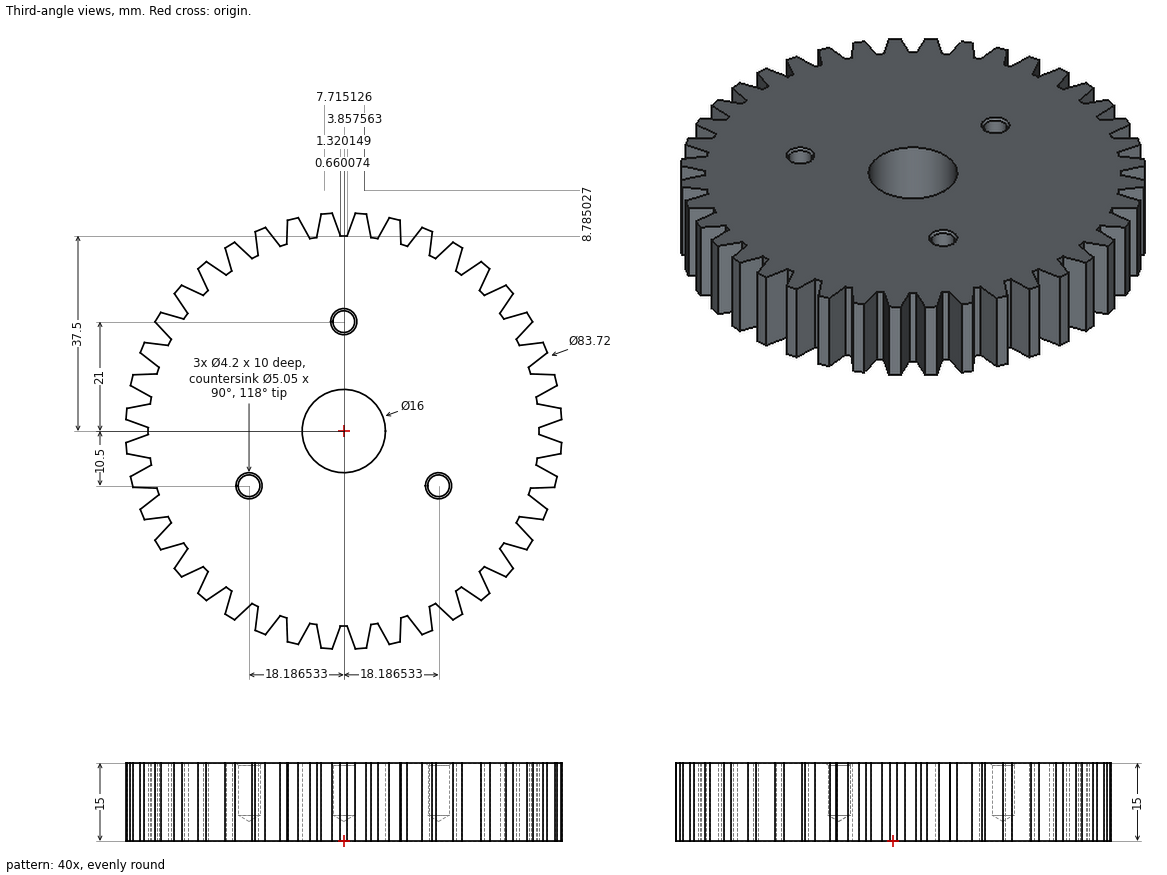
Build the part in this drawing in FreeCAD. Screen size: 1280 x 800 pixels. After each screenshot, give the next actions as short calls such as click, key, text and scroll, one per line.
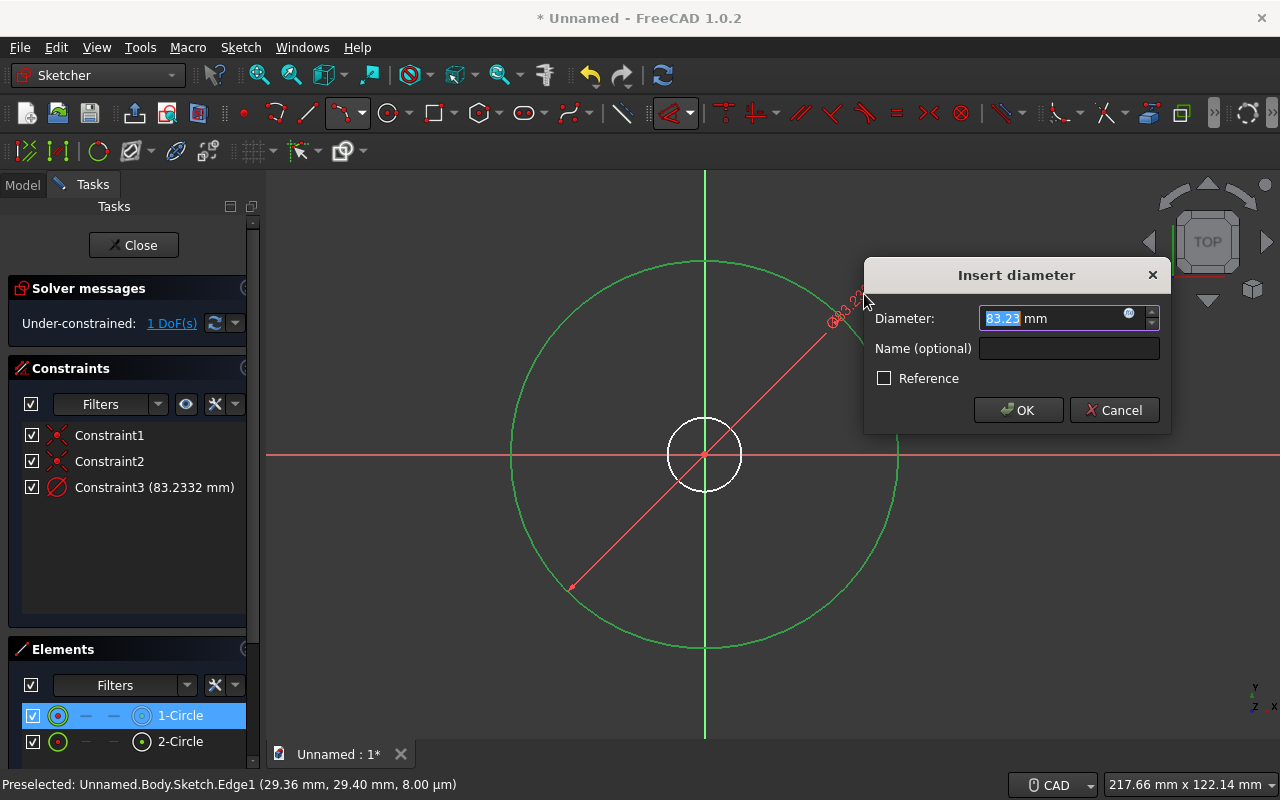
text(83.72)
key(Return)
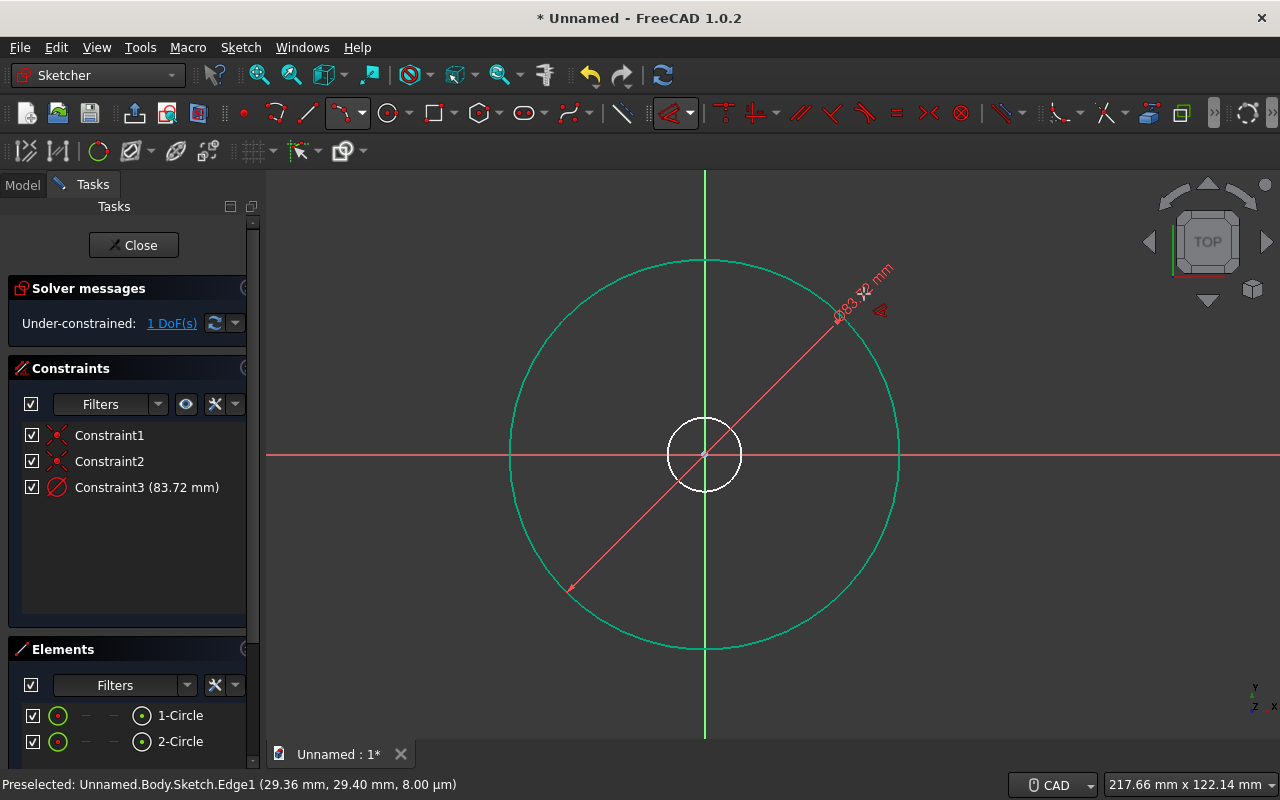
click(731, 429)
click(754, 407)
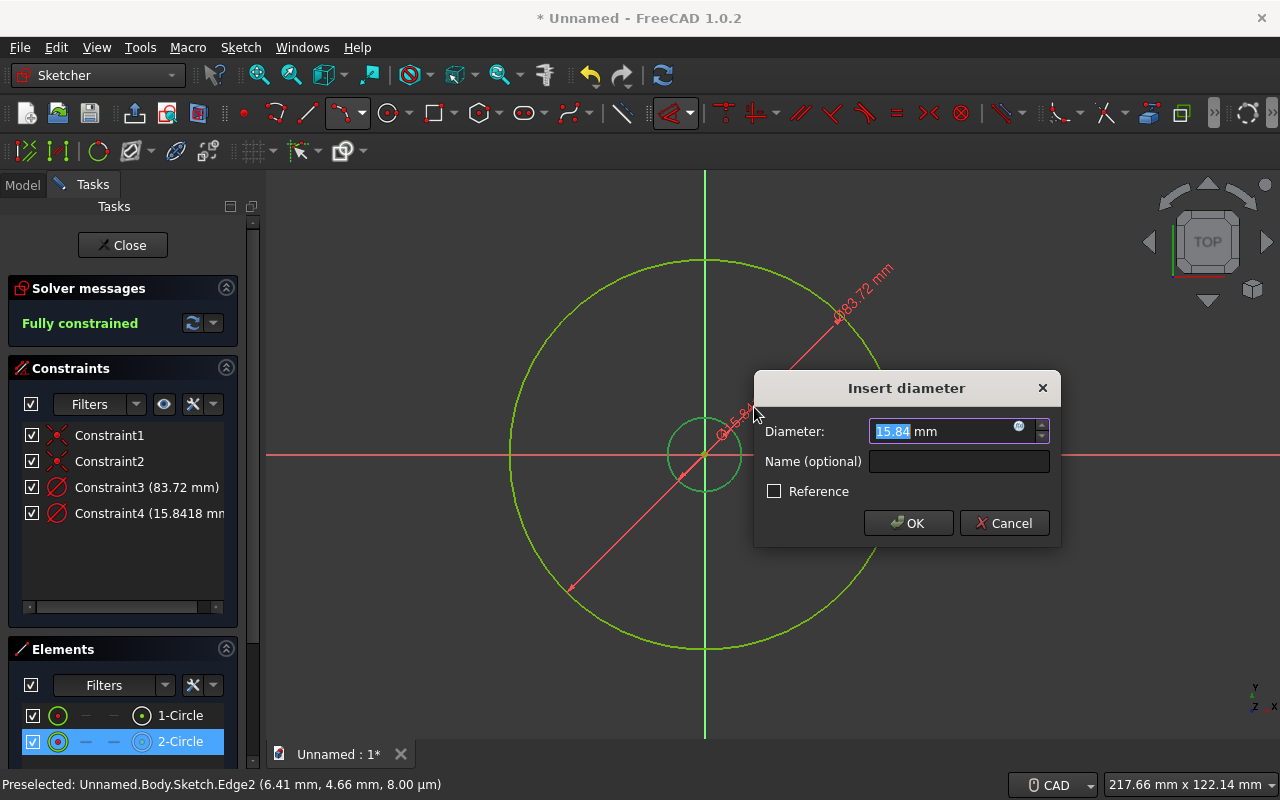
text(16)
key(Return)
key(Escape)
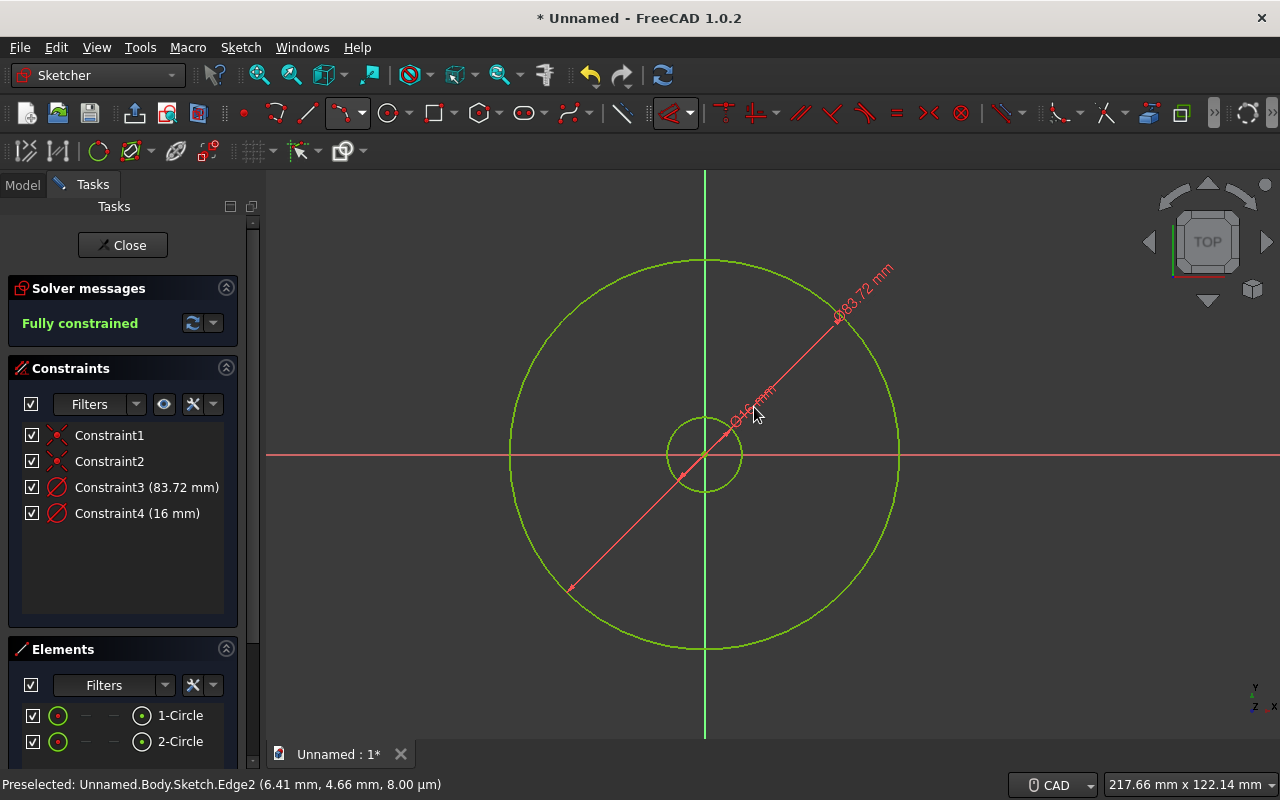
click(123, 245)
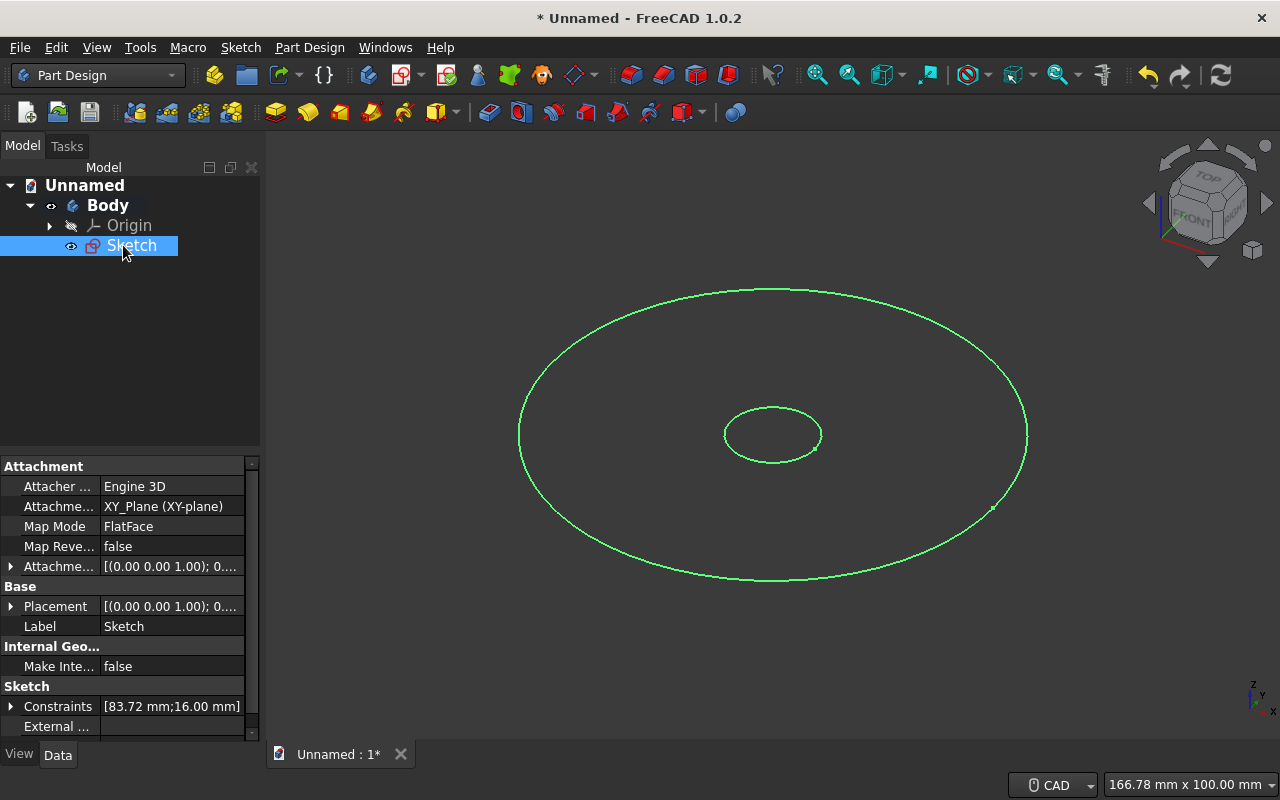
click(276, 112)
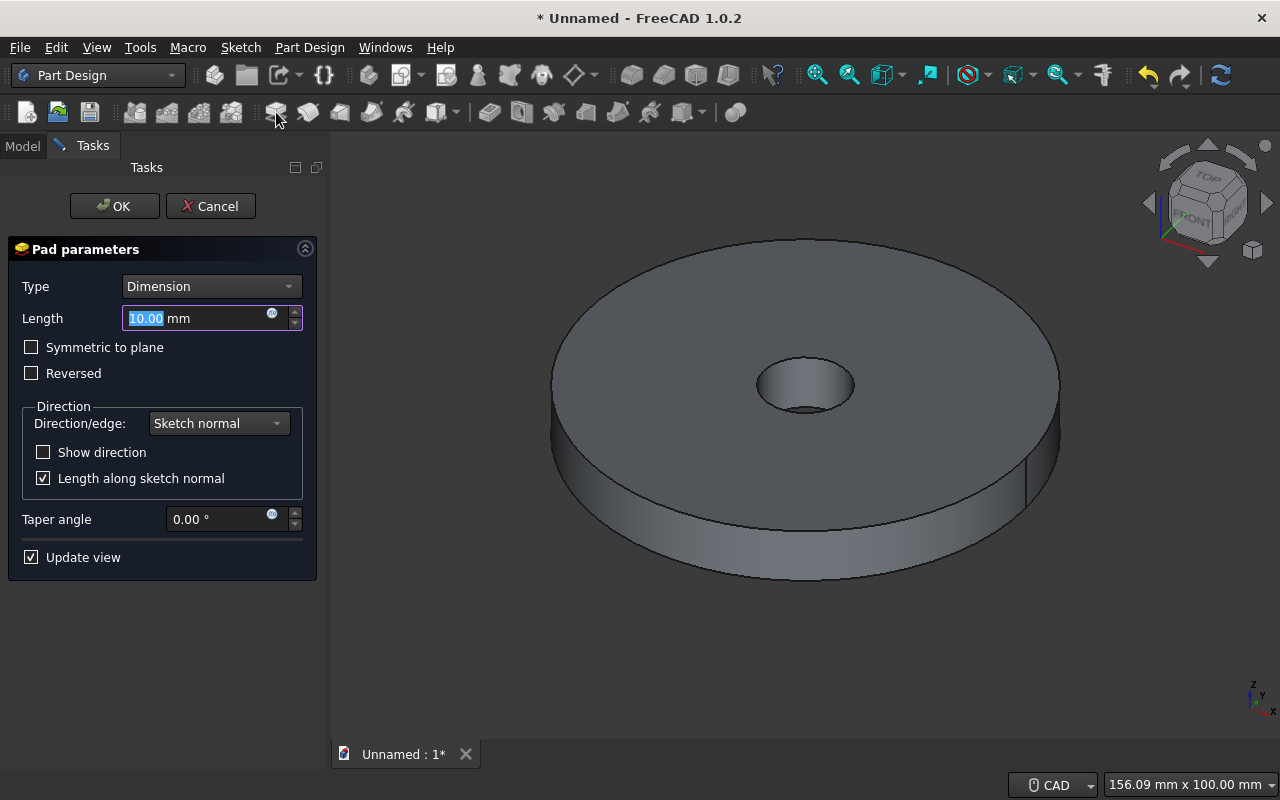
text(15)
key(Tab)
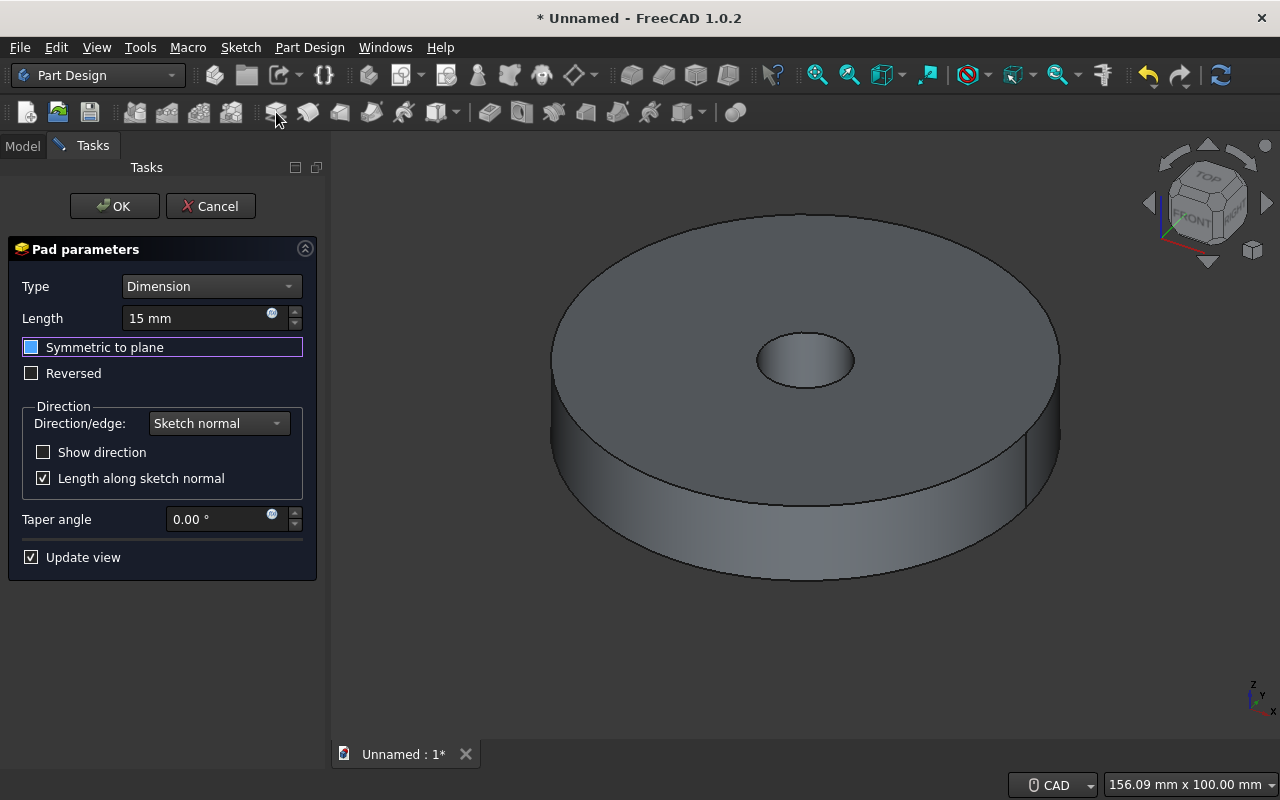
click(115, 206)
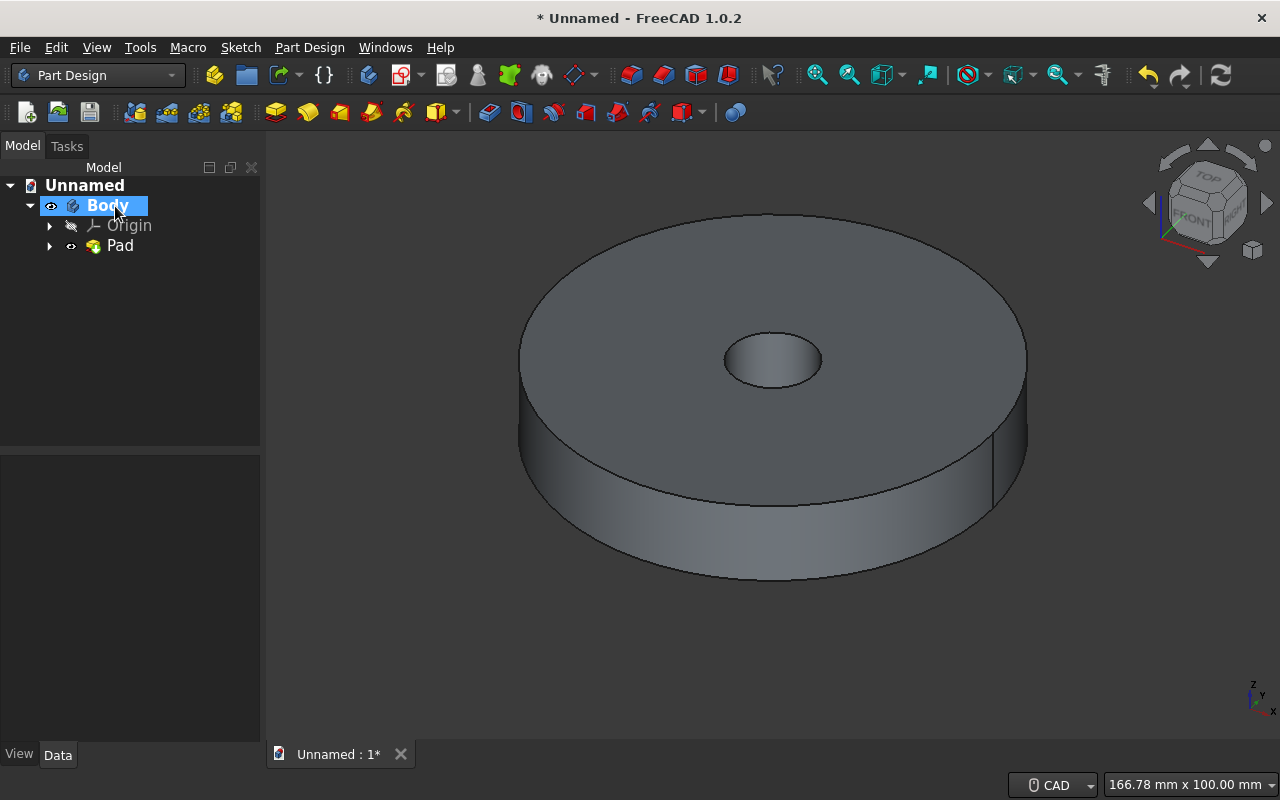
click(846, 287)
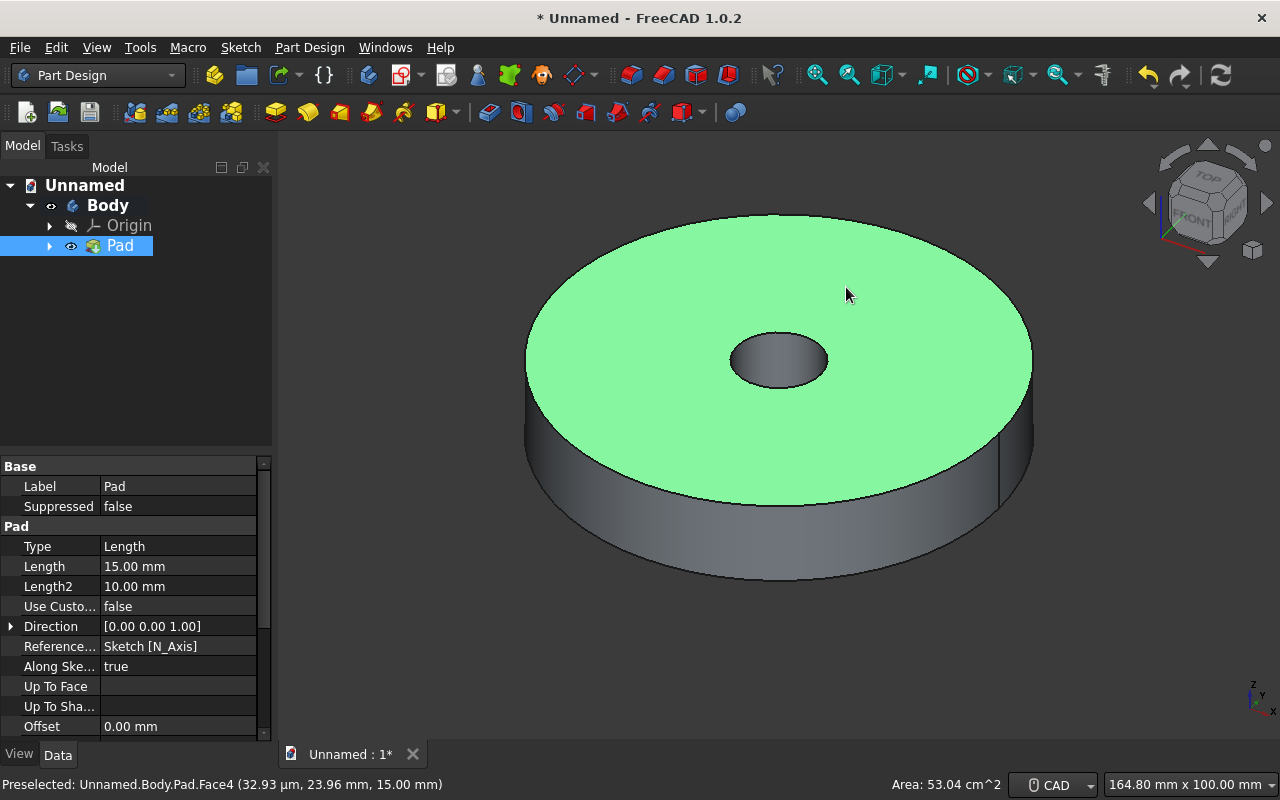
click(402, 76)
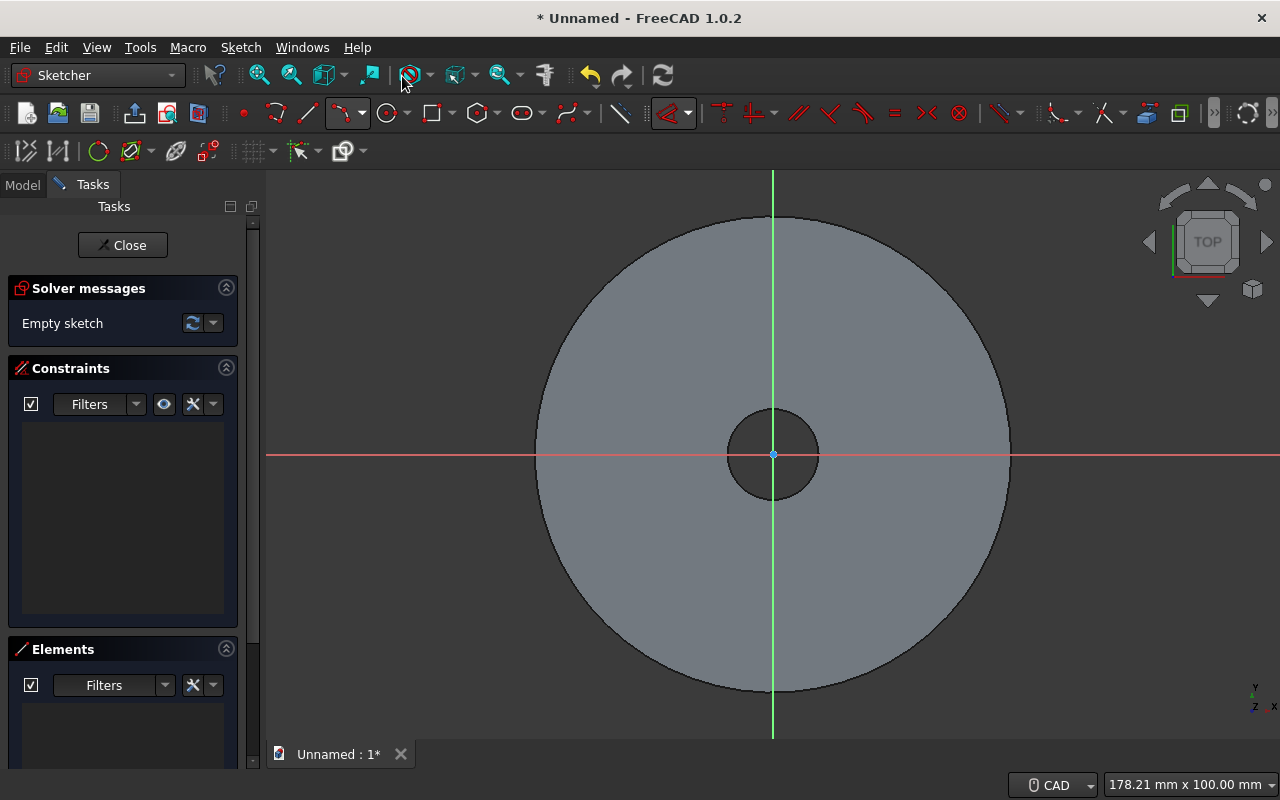
scroll(856, 388, up, 3)